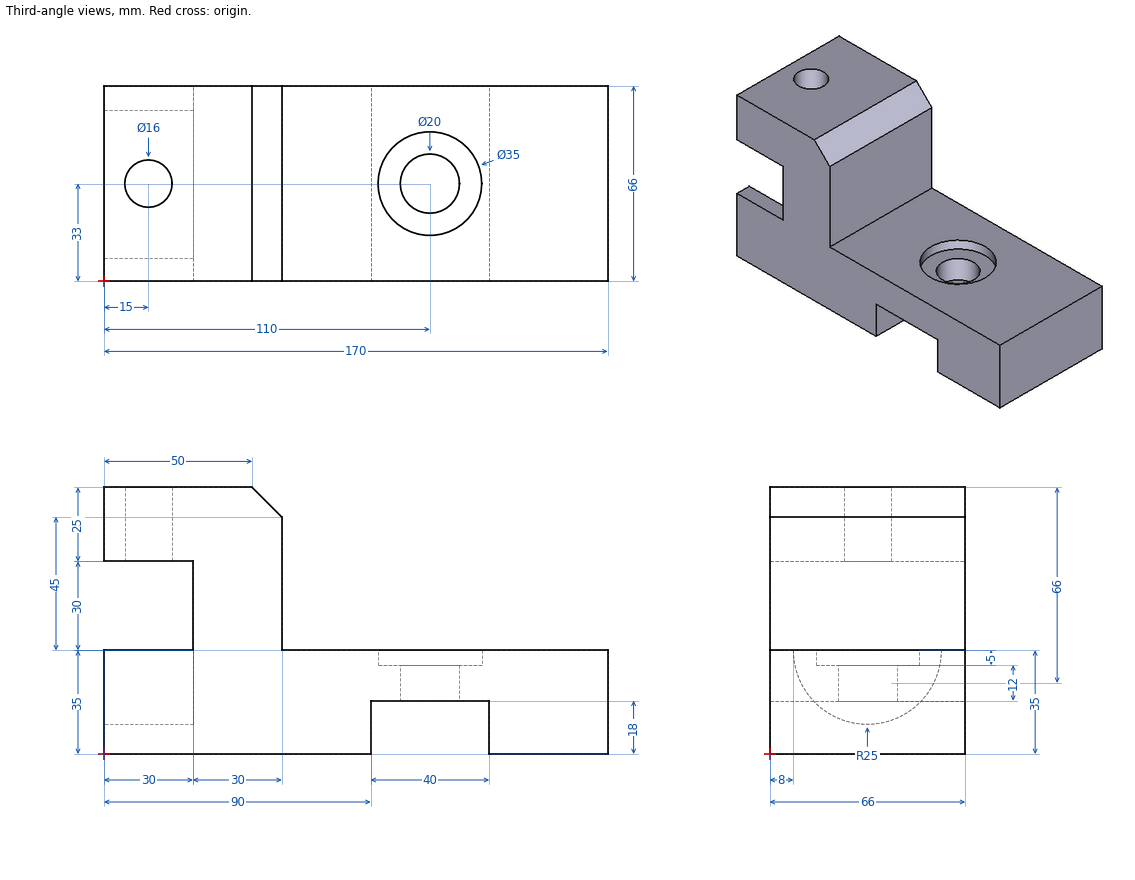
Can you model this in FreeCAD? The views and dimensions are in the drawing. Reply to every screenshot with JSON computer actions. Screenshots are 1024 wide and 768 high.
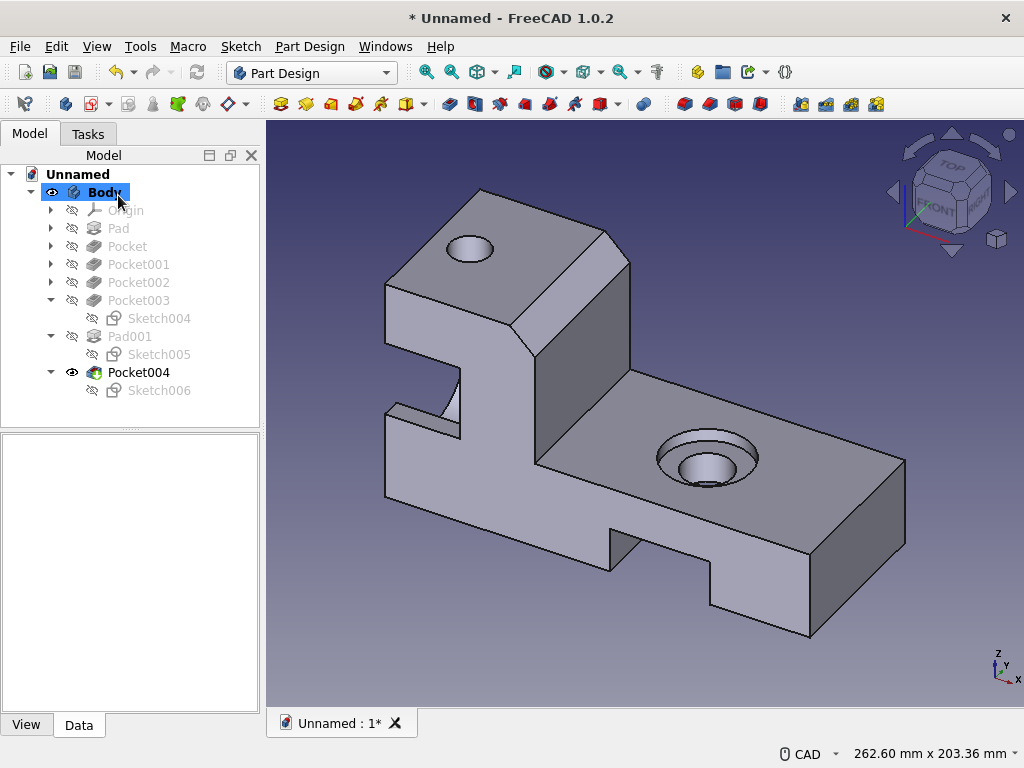
{"action": "key", "text": "0"}